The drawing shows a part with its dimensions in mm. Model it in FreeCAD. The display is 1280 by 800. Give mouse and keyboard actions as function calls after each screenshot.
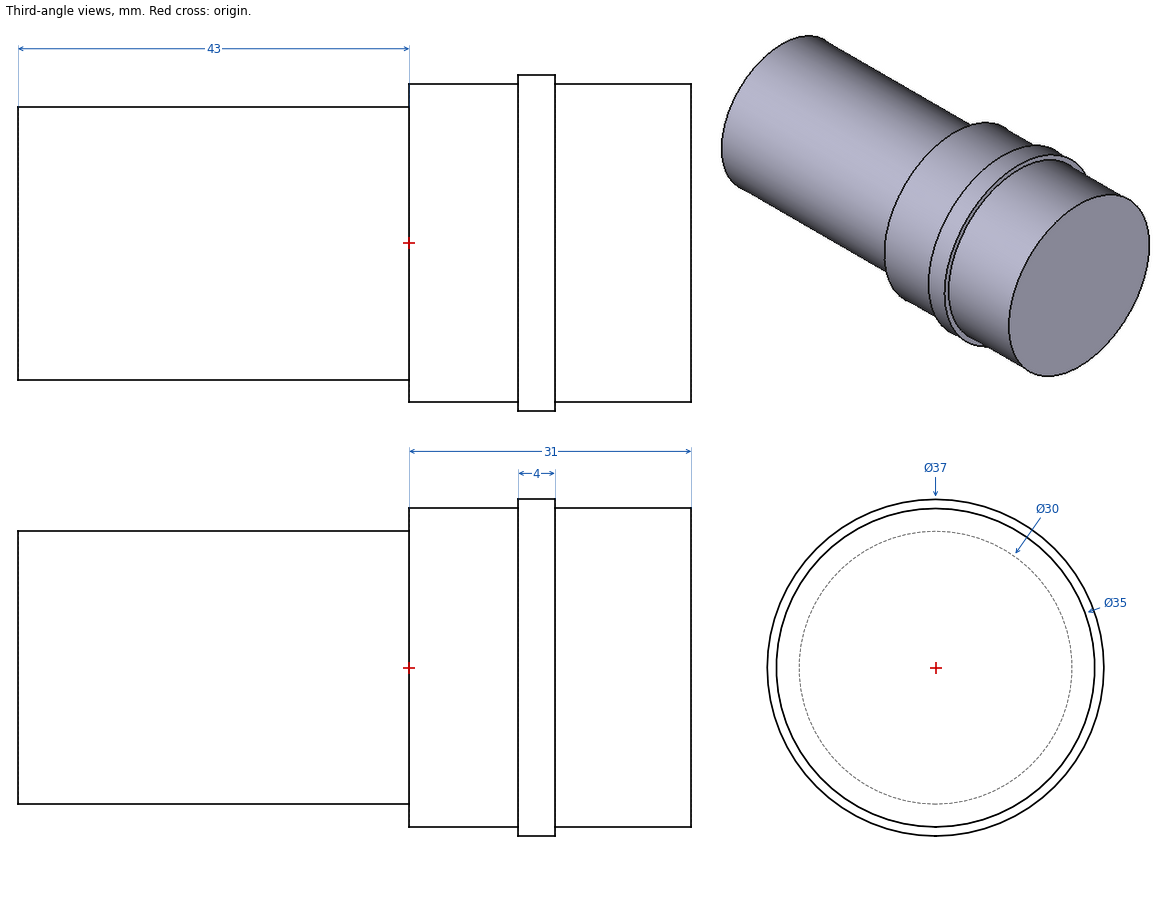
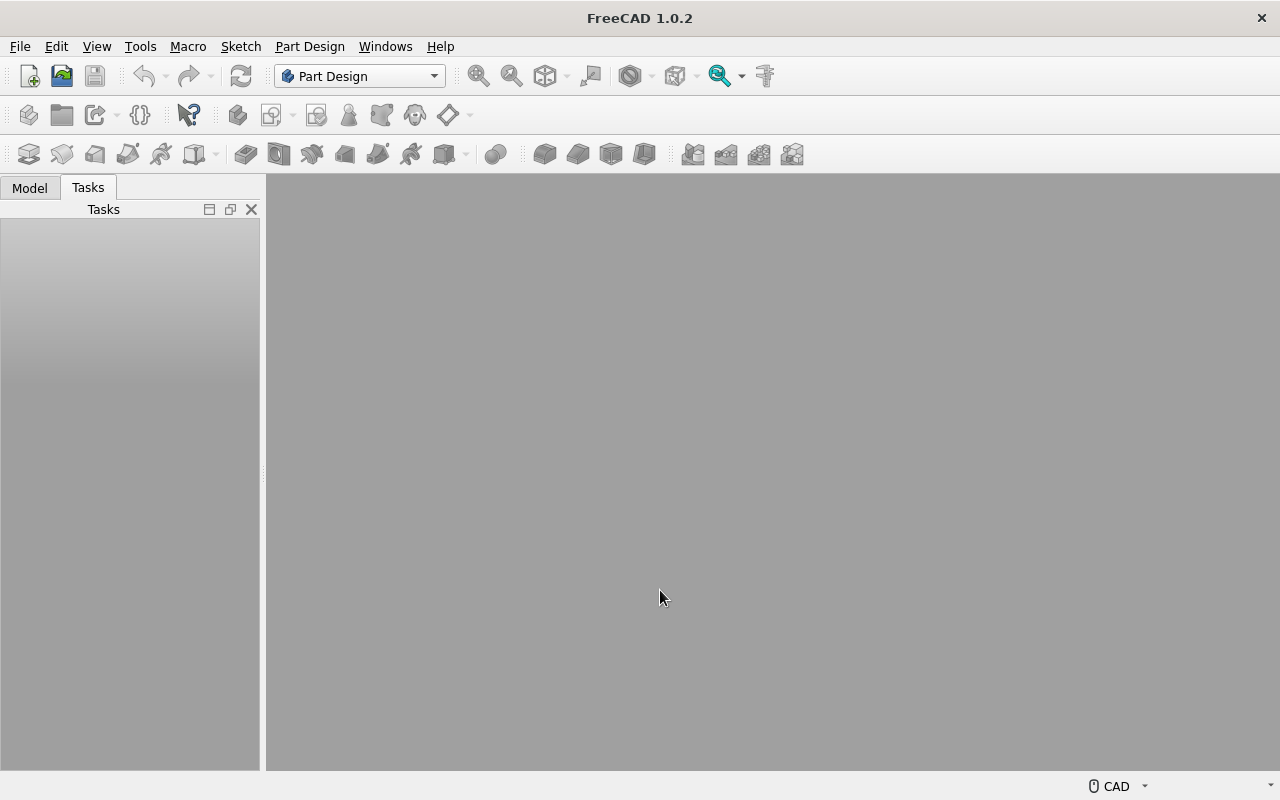
click(29, 76)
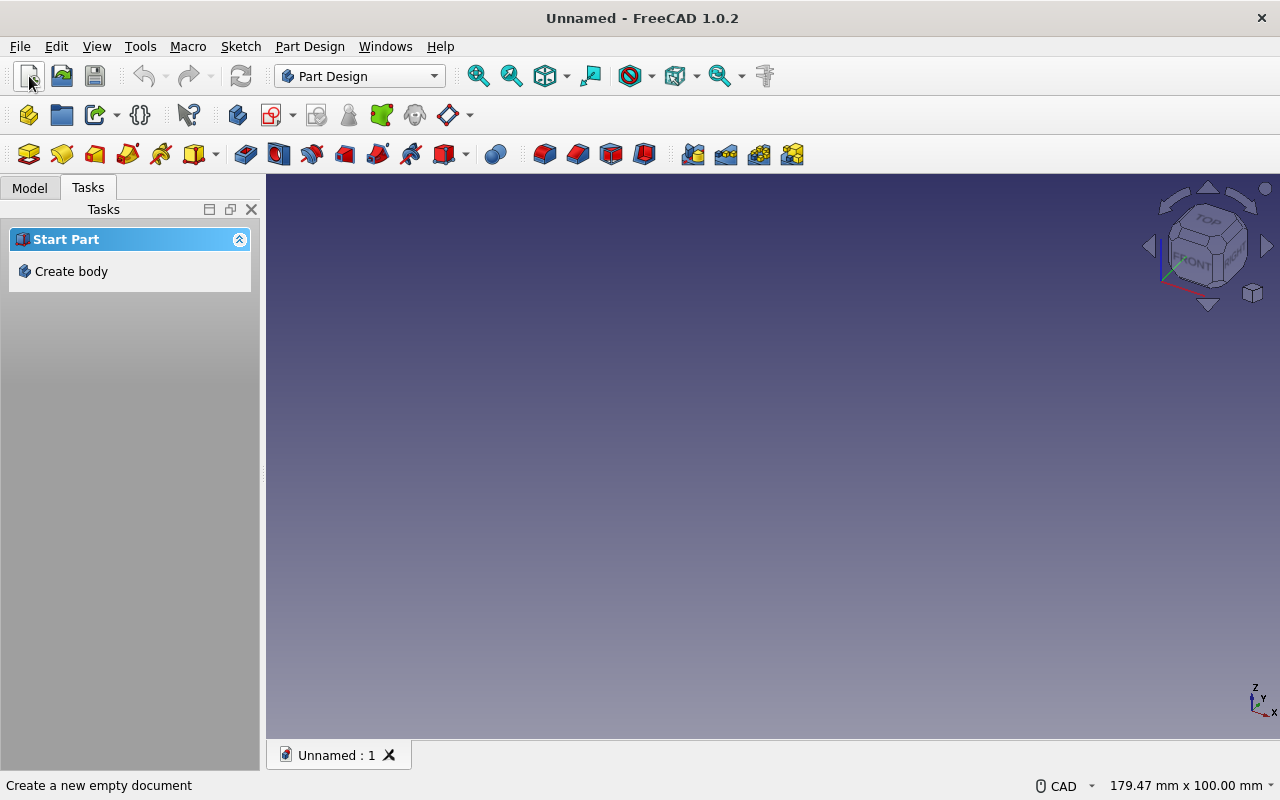
click(270, 116)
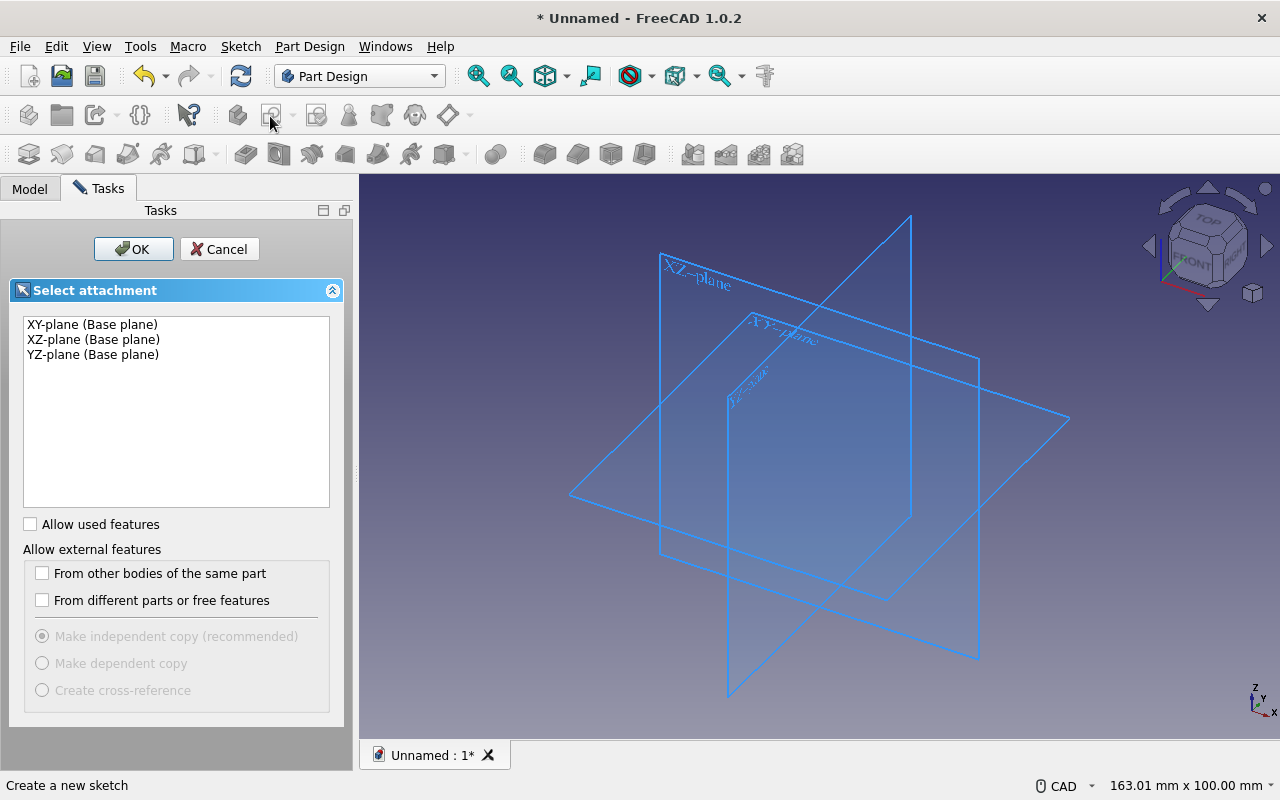
click(84, 354)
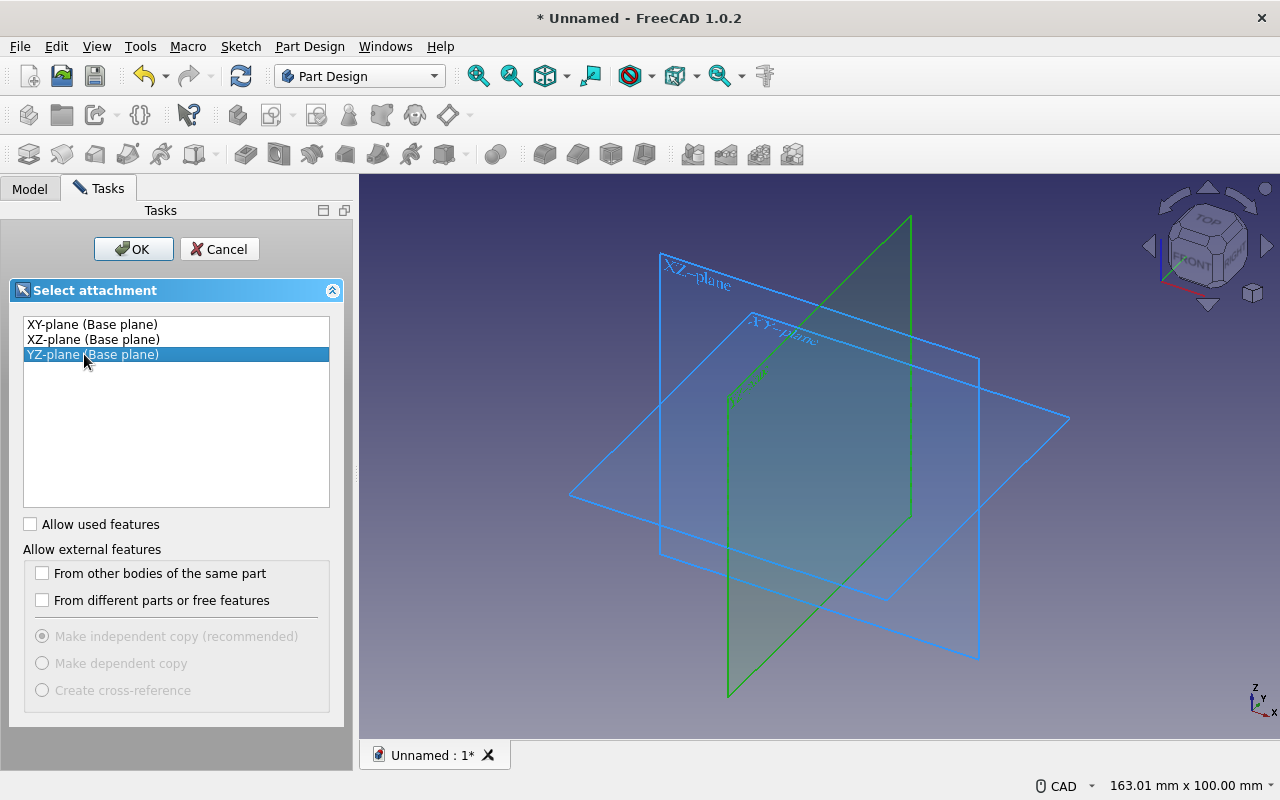
click(134, 249)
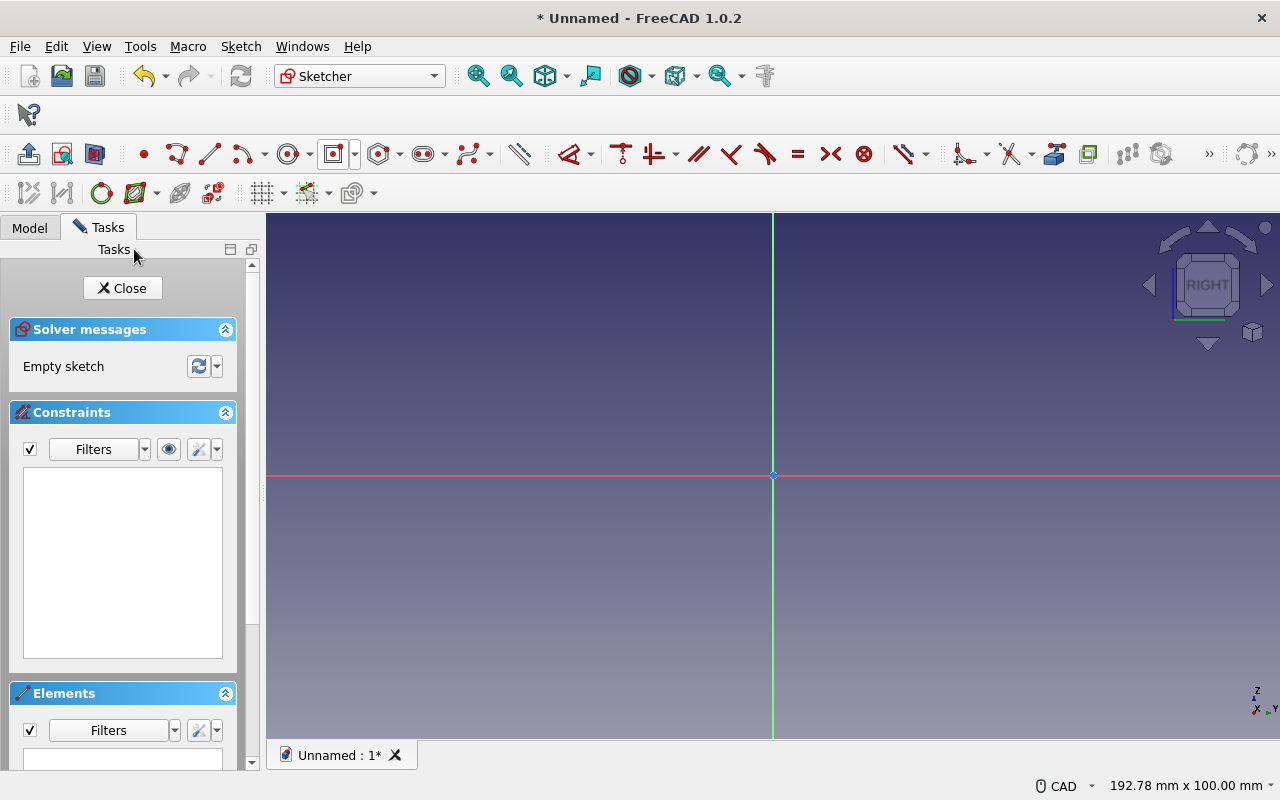
scroll(856, 476, up, 3)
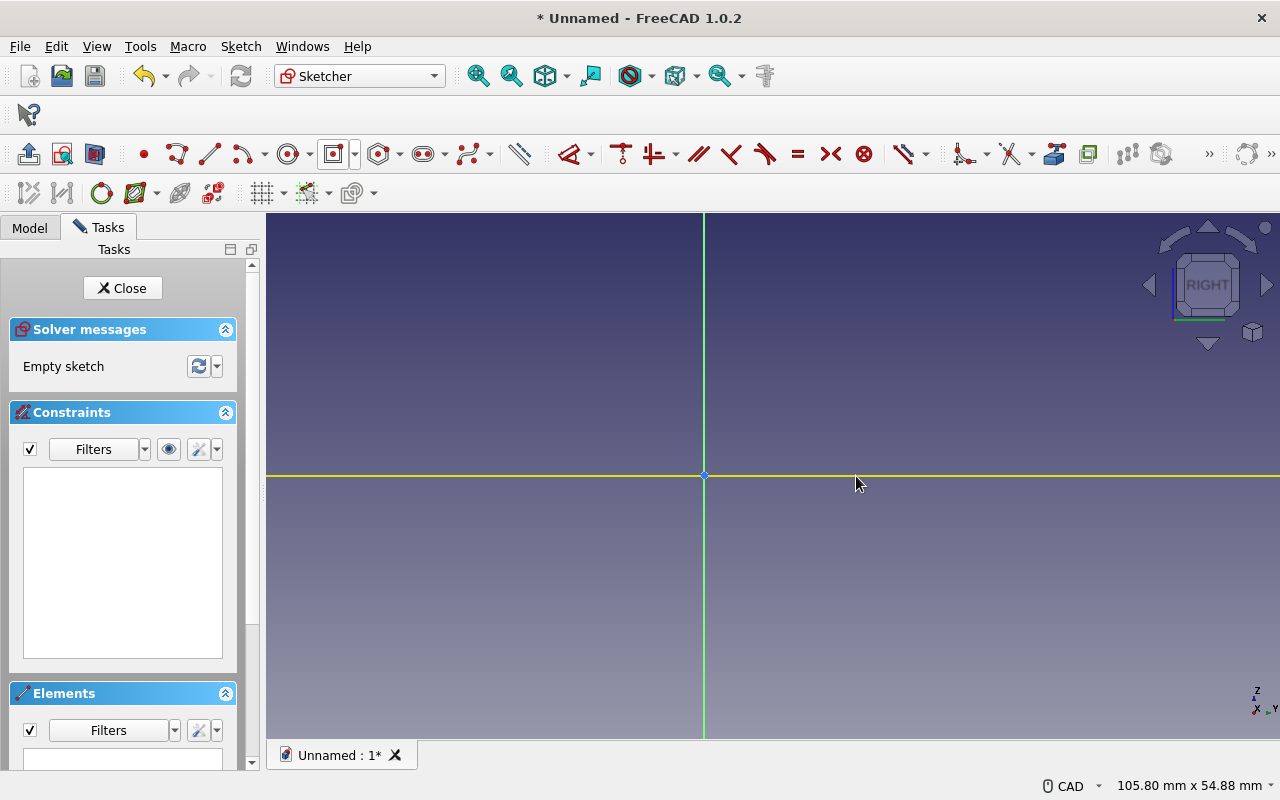
click(288, 154)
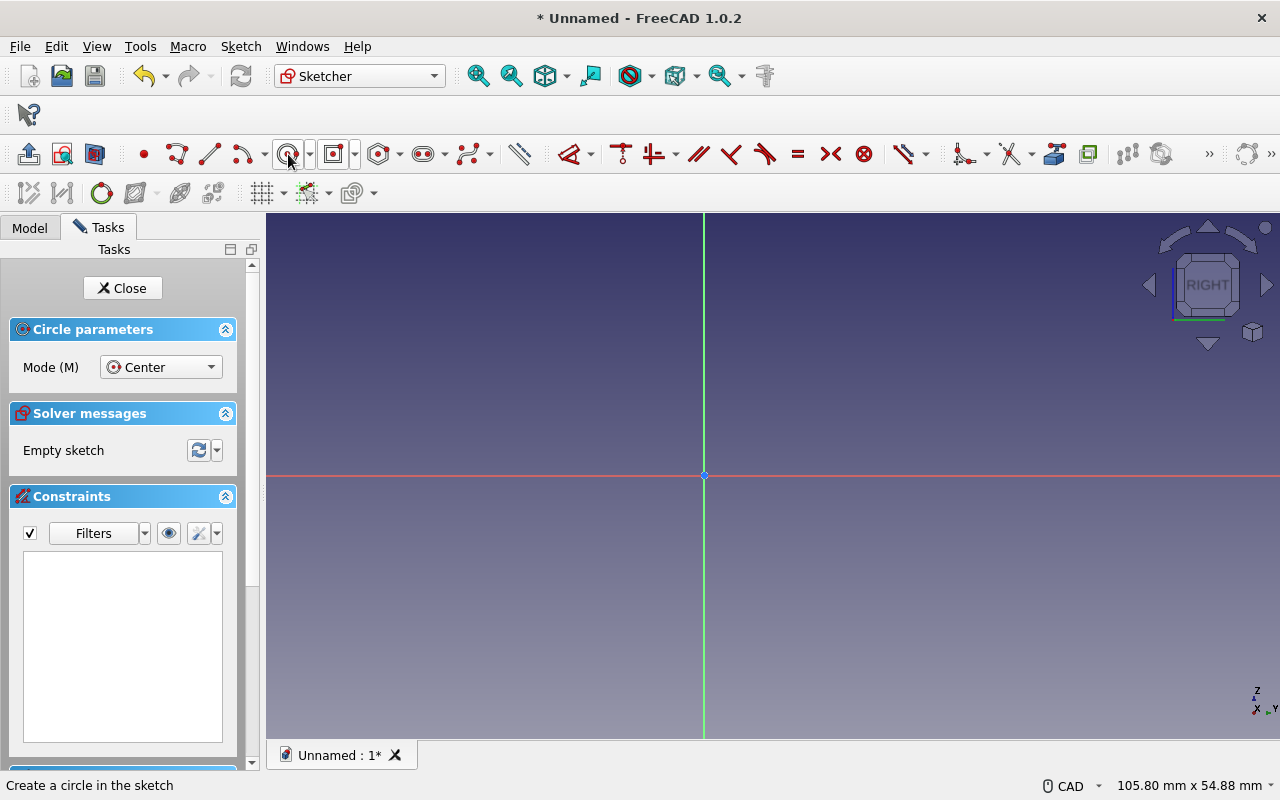
click(704, 476)
click(823, 357)
key(Escape)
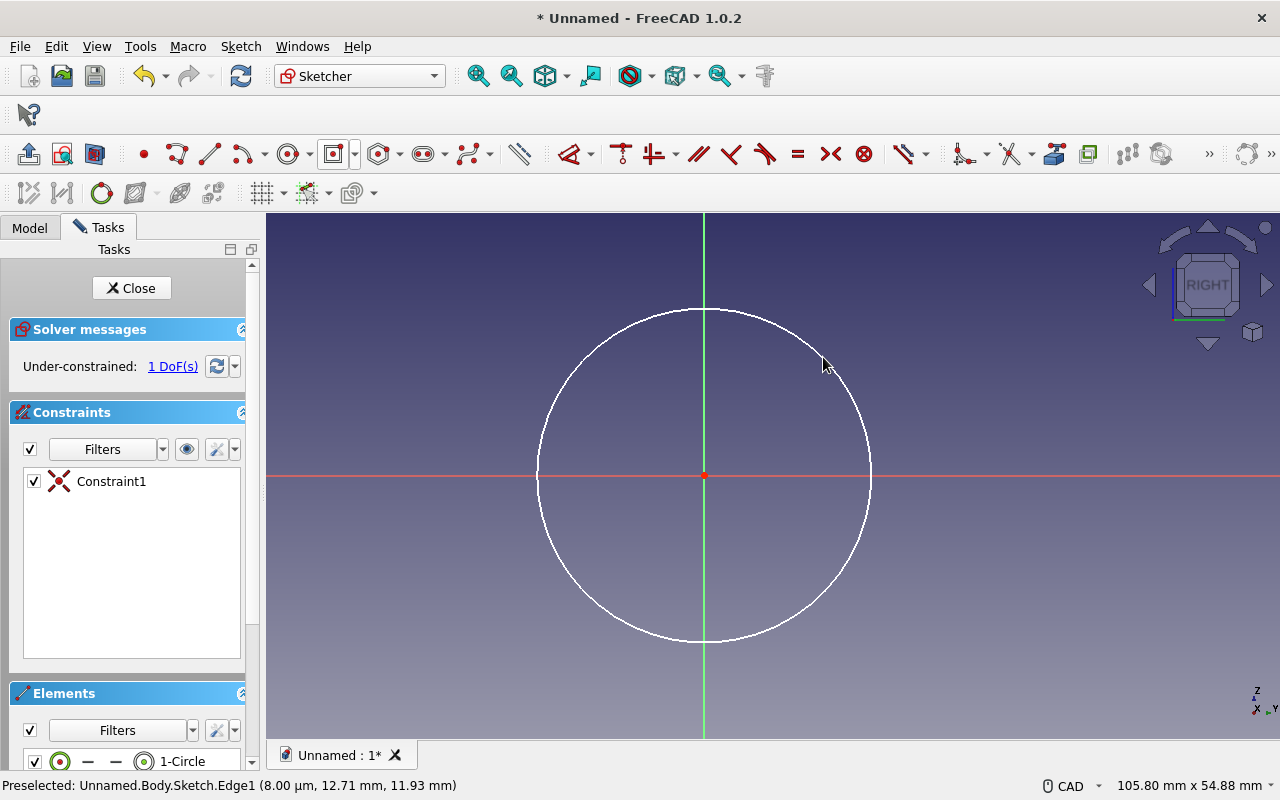
click(568, 154)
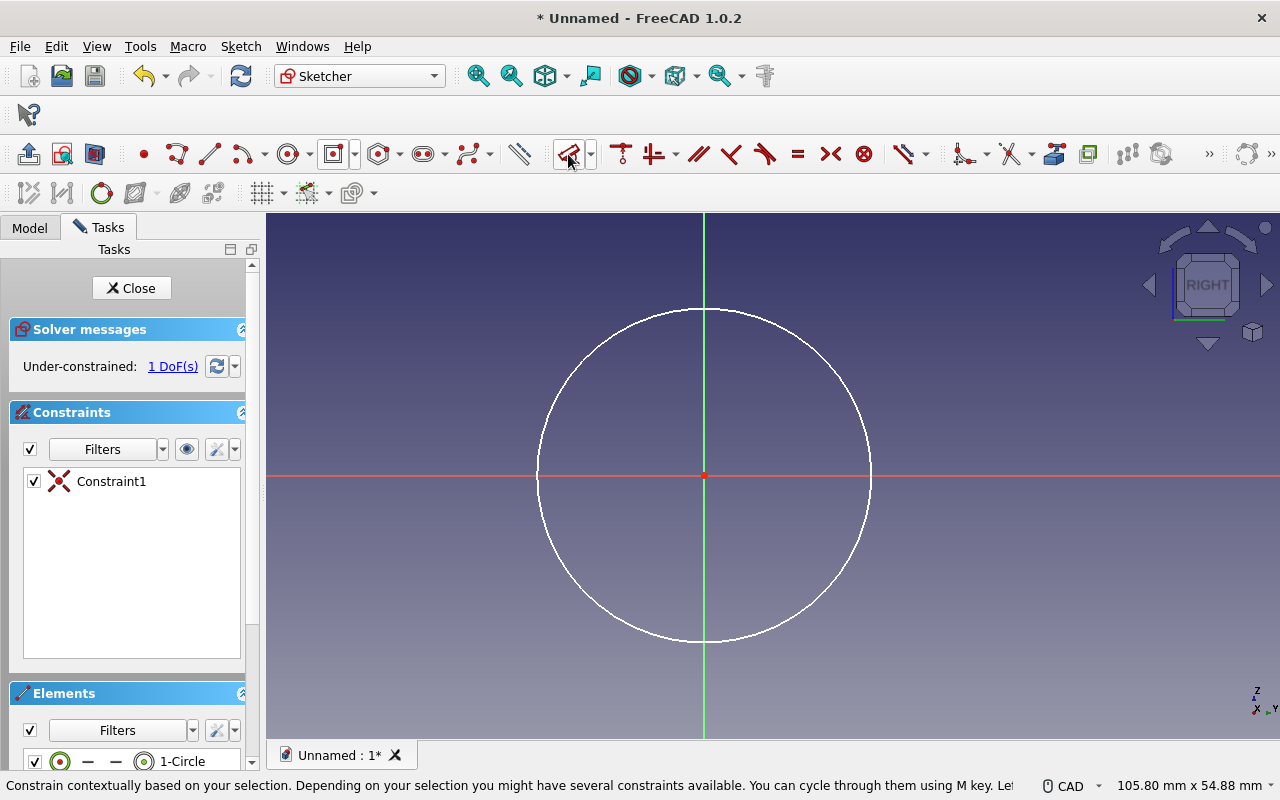
click(822, 357)
click(845, 334)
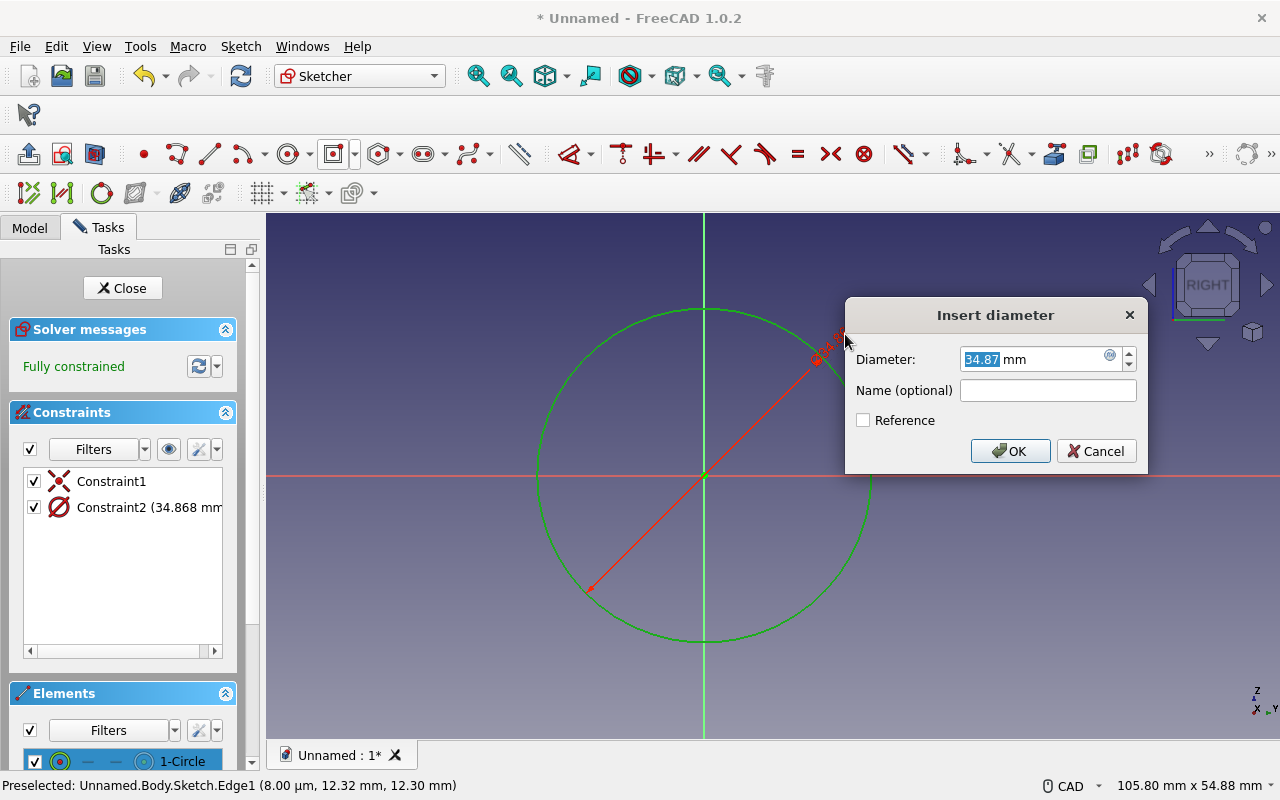
text(35)
key(Return)
key(Escape)